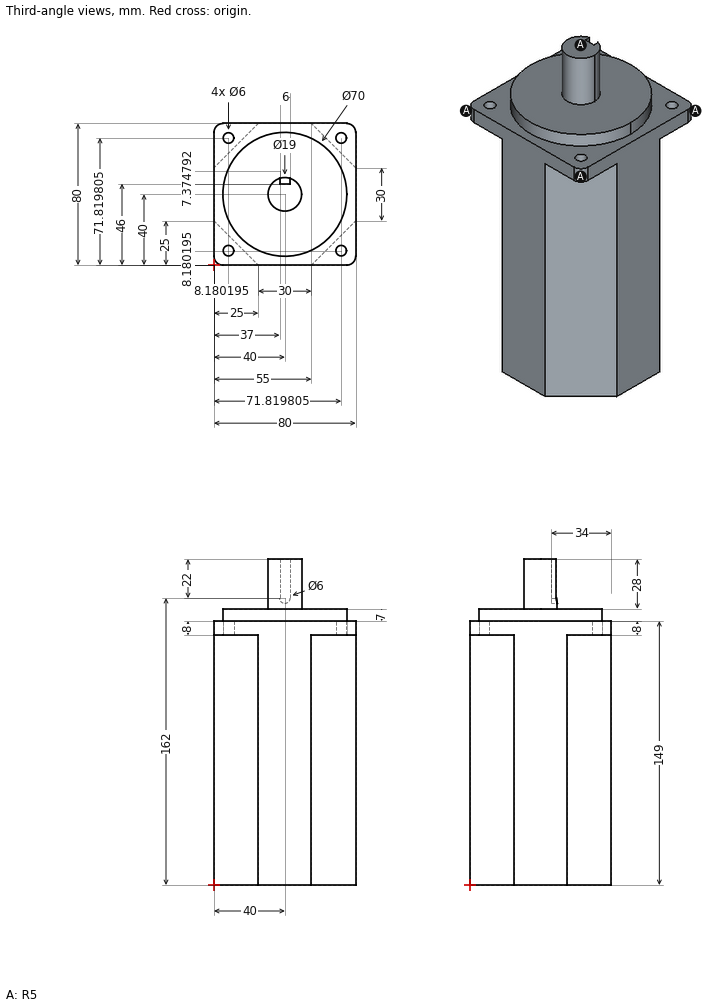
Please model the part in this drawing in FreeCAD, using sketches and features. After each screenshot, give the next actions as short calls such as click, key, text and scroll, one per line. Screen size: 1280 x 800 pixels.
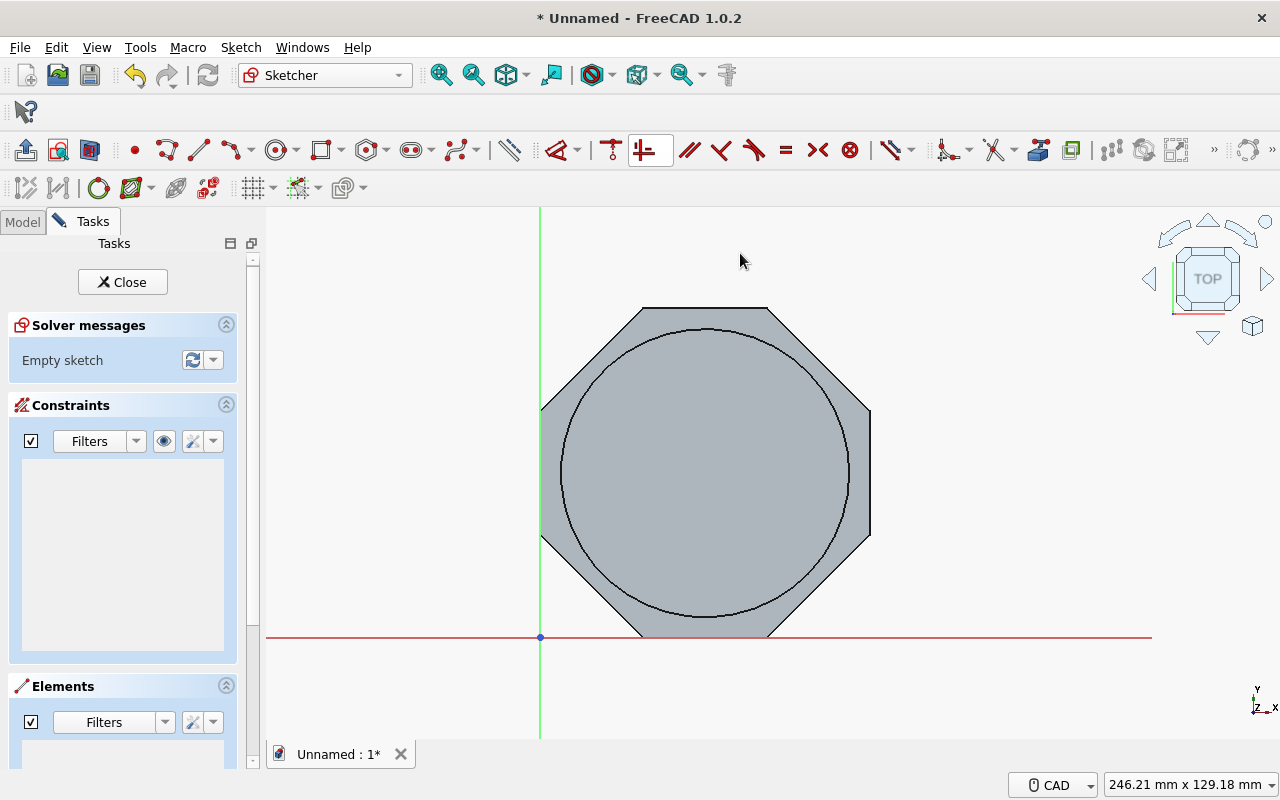
key(g)
key(r)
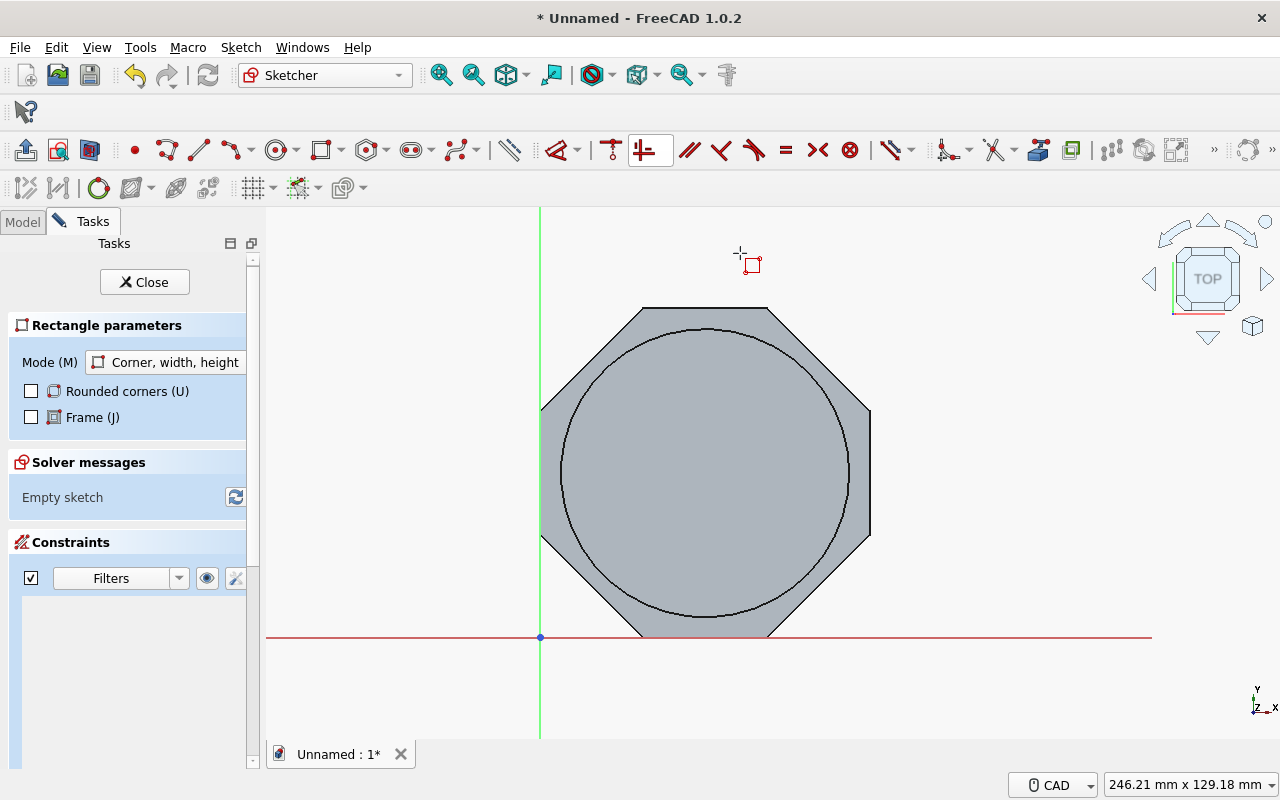
click(540, 638)
click(870, 308)
key(Escape)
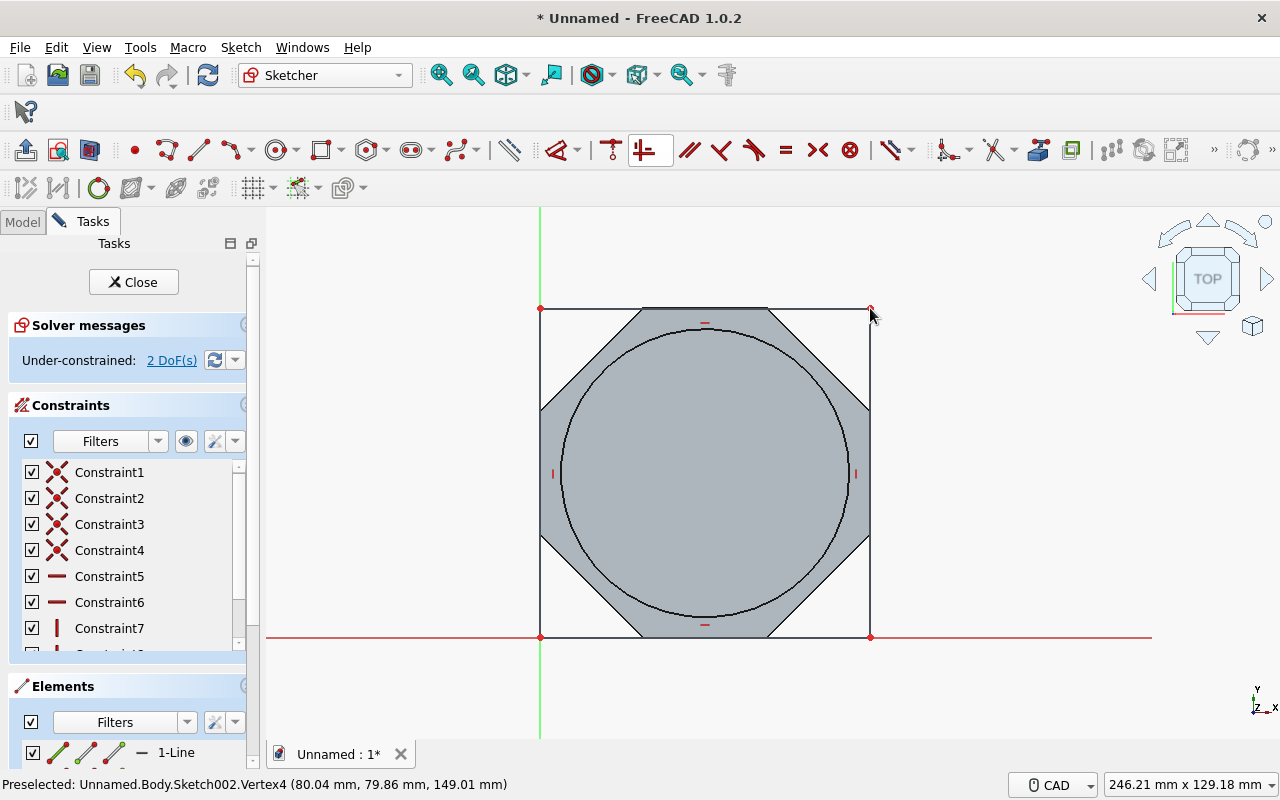
click(556, 150)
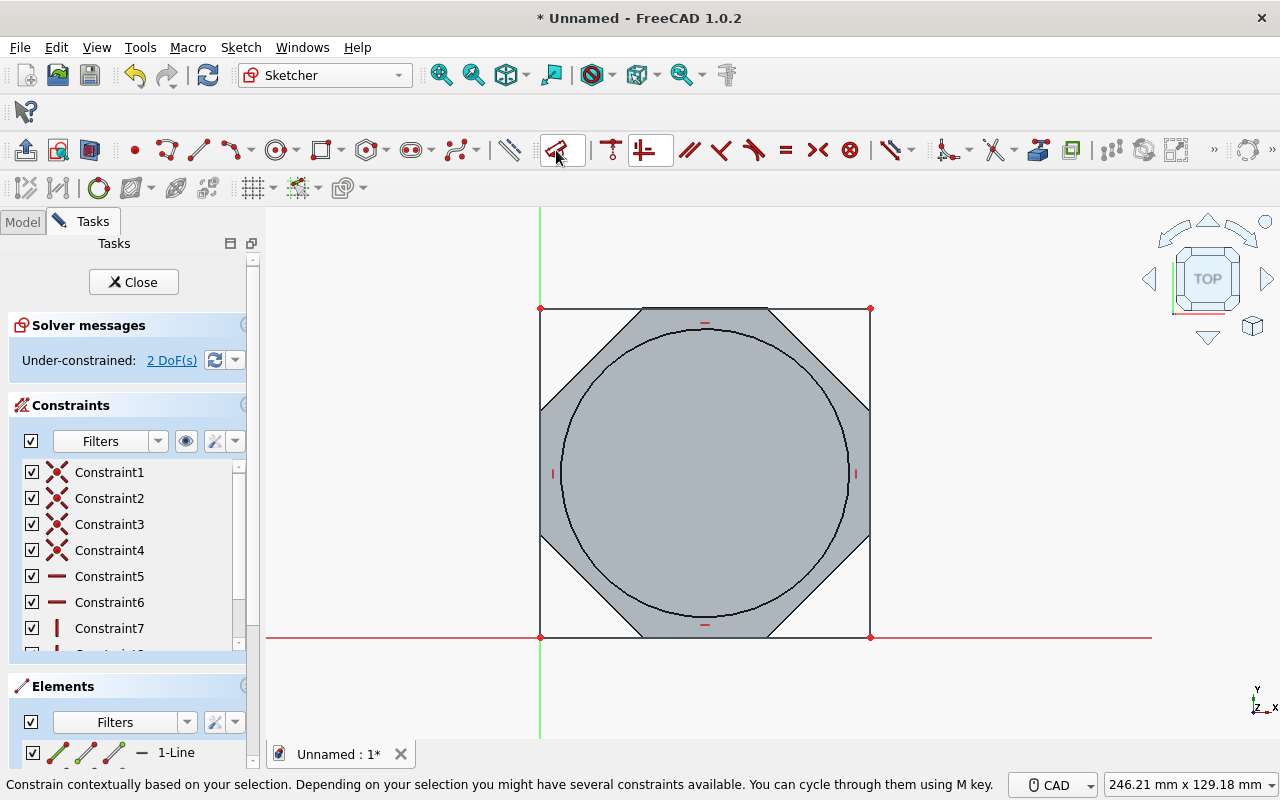
click(639, 638)
click(705, 672)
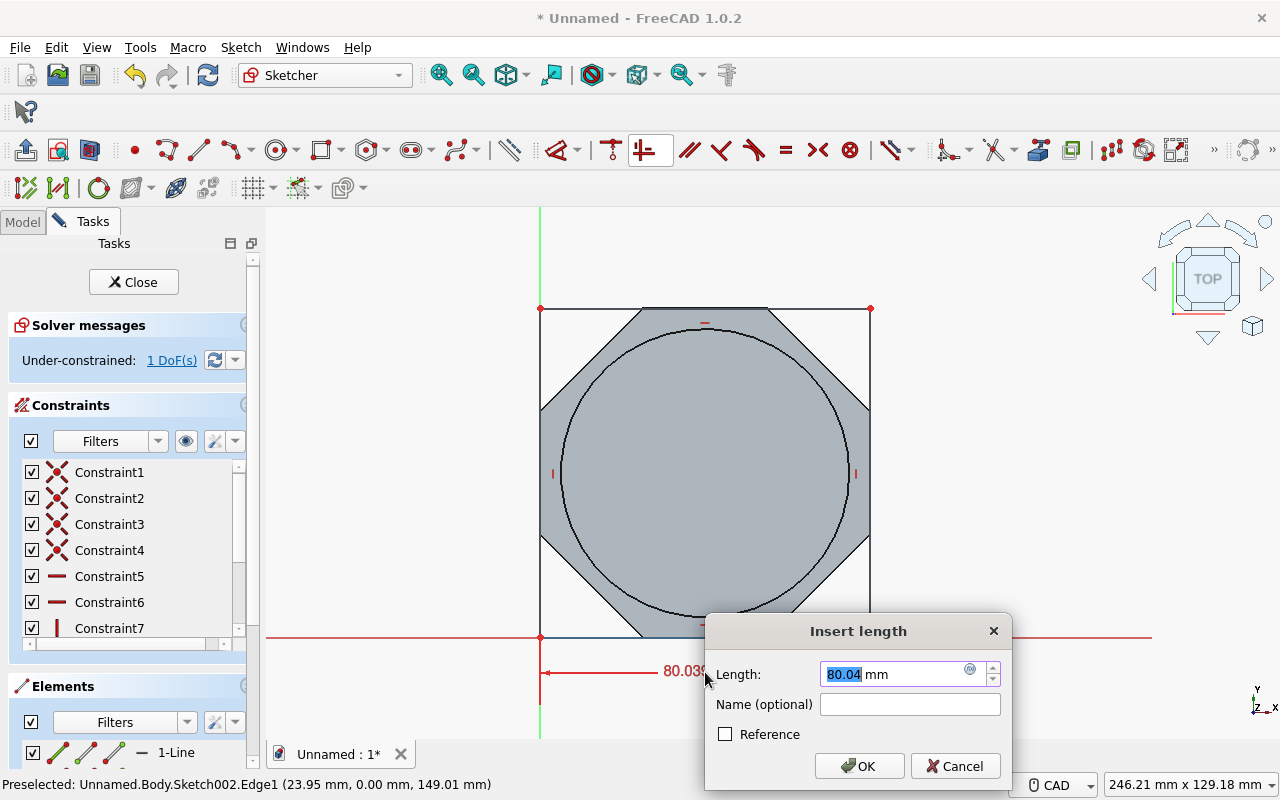
text(80)
key(Return)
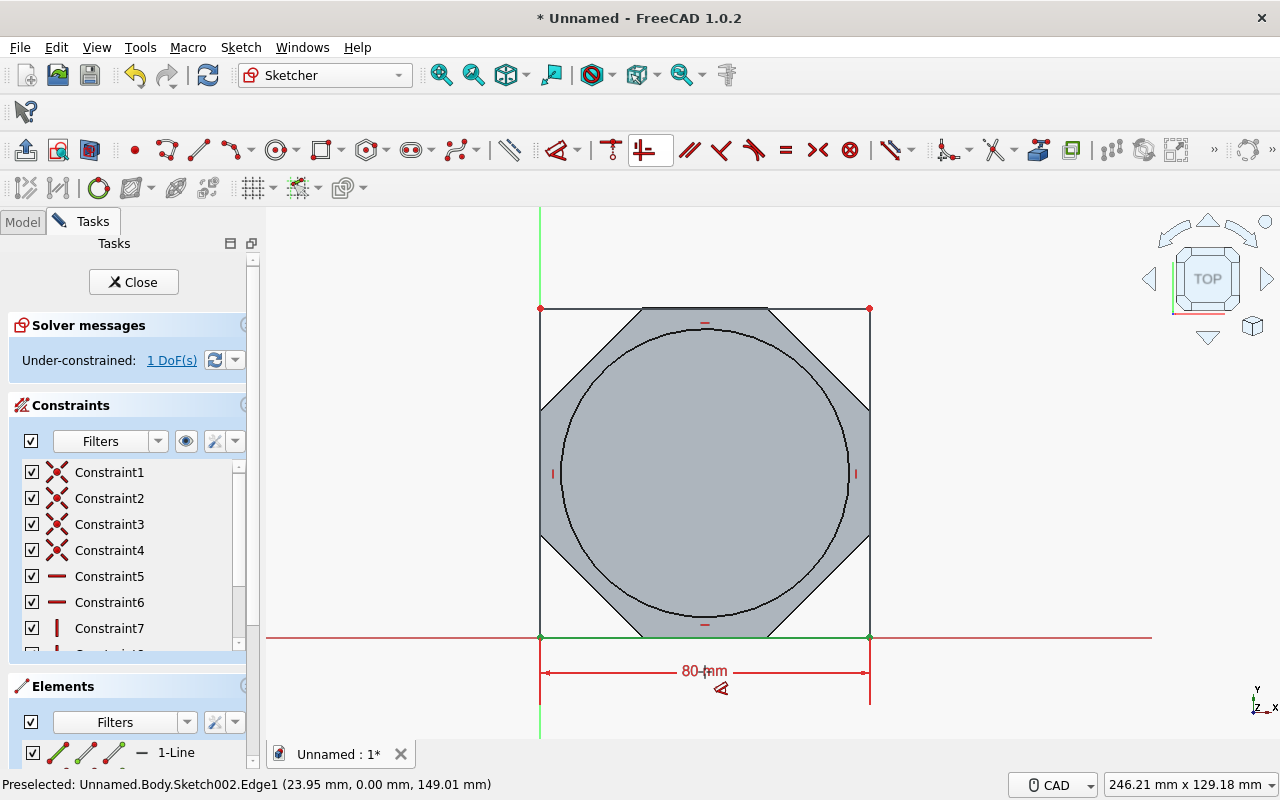
click(870, 539)
click(904, 473)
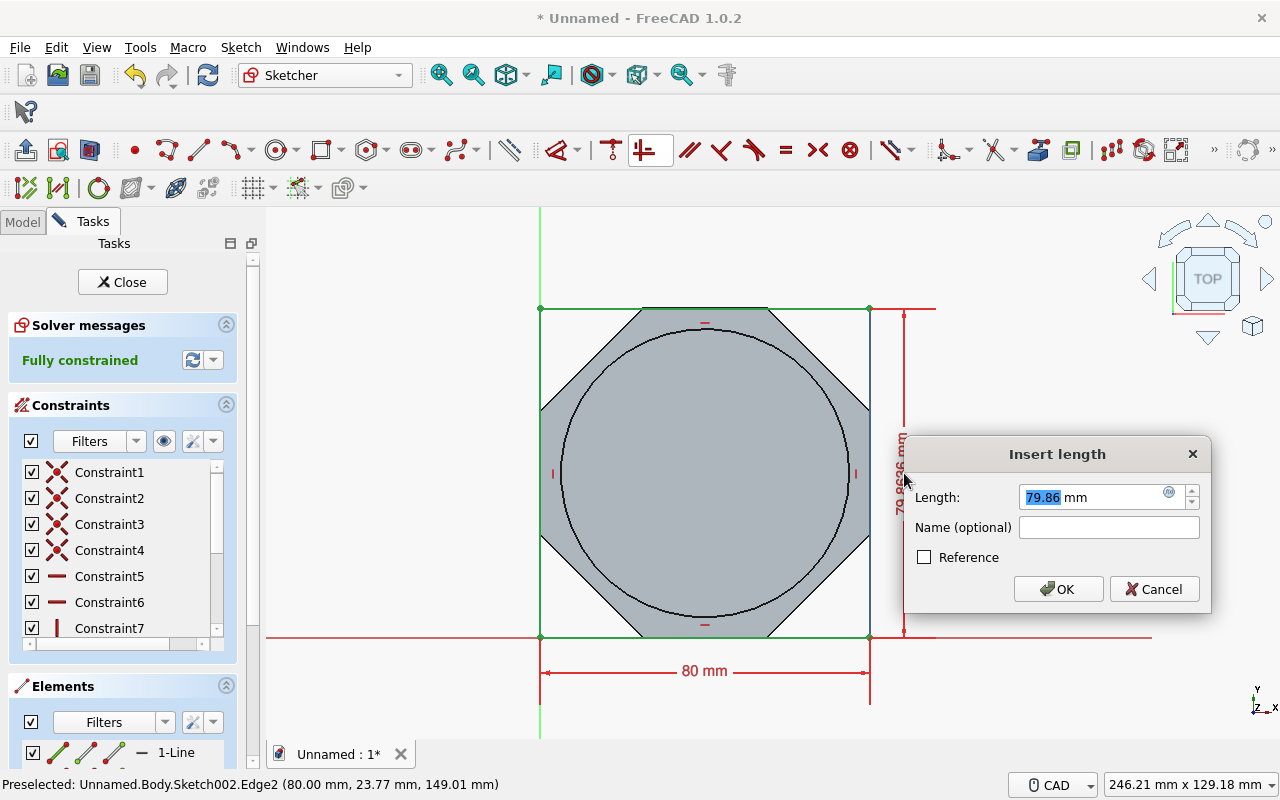
text(80)
key(Return)
key(Escape)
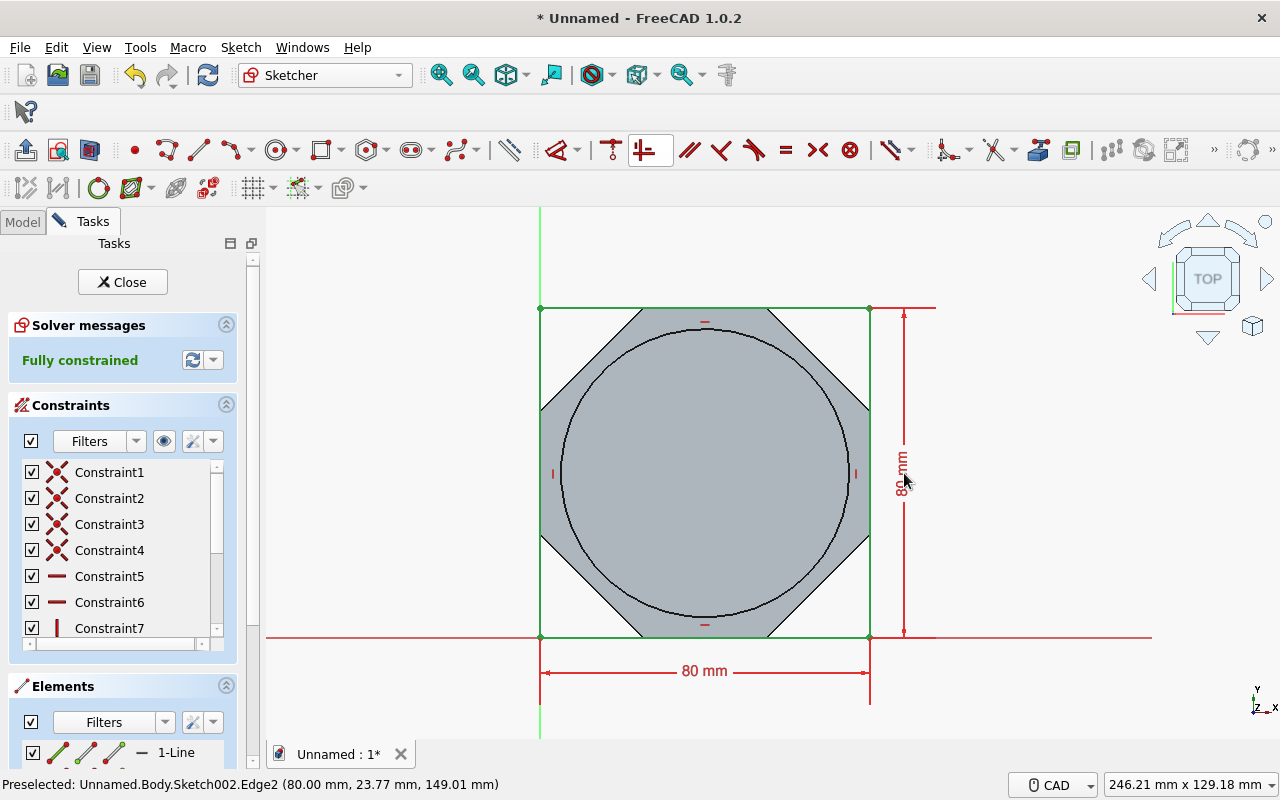
click(123, 282)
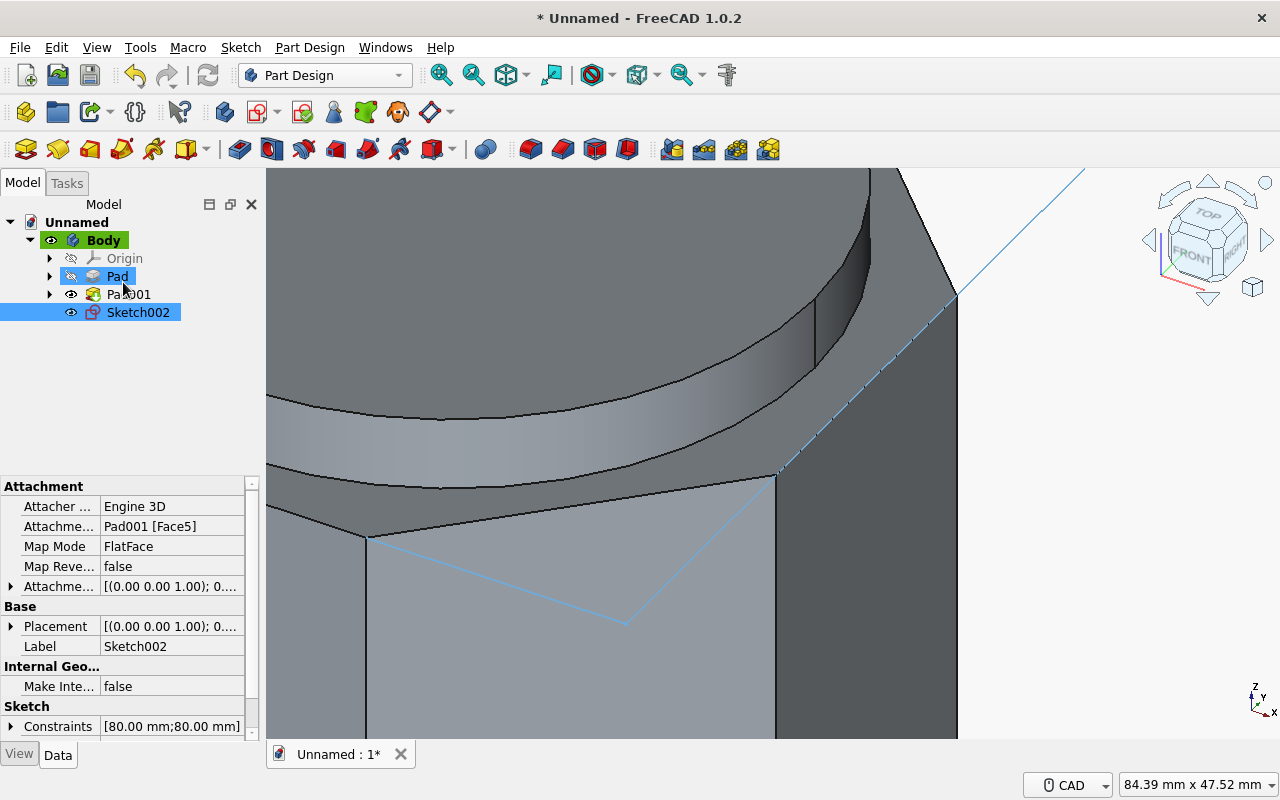
click(26, 150)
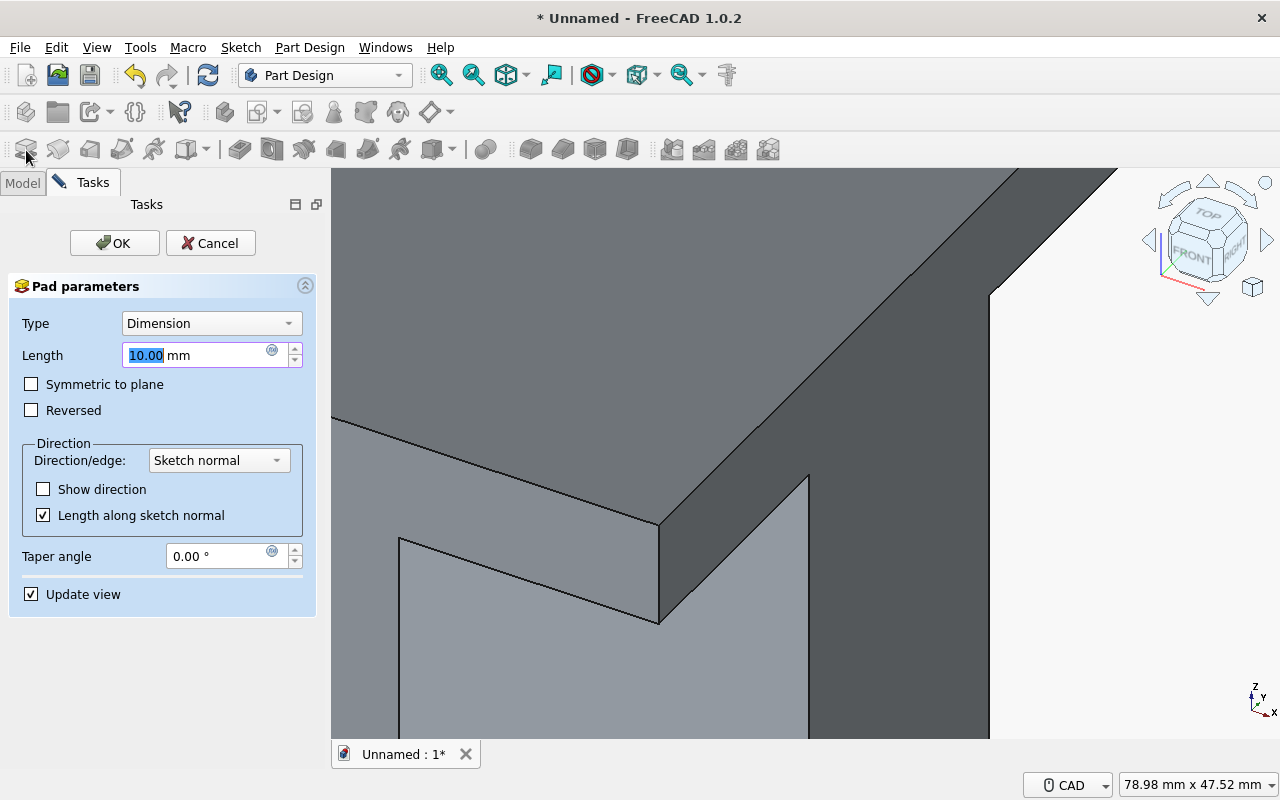
text(8)
key(Tab)